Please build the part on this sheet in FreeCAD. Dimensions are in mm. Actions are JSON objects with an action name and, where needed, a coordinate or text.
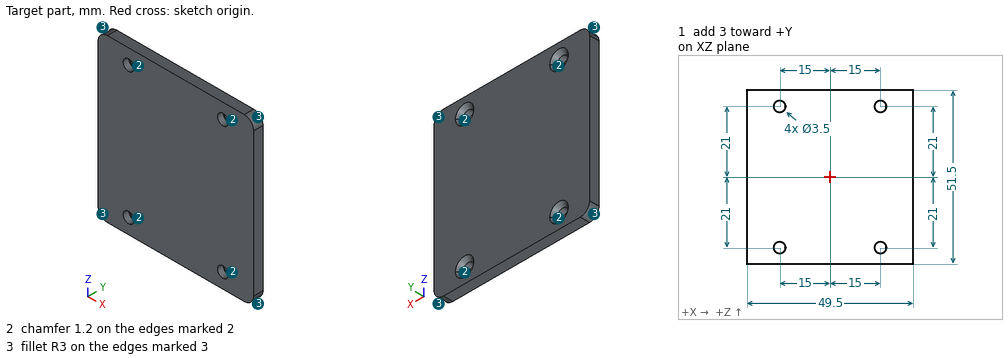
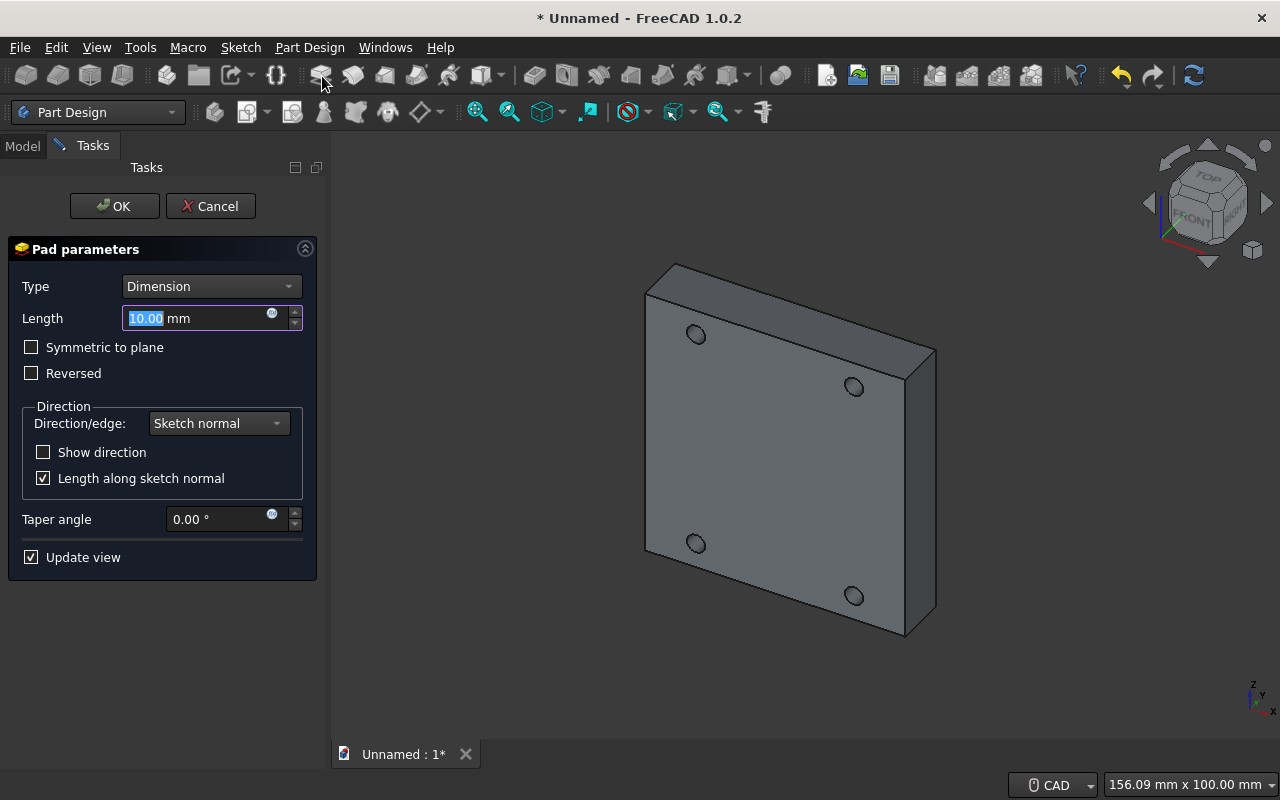
{"action": "type", "text": "3"}
{"action": "key", "text": "Tab"}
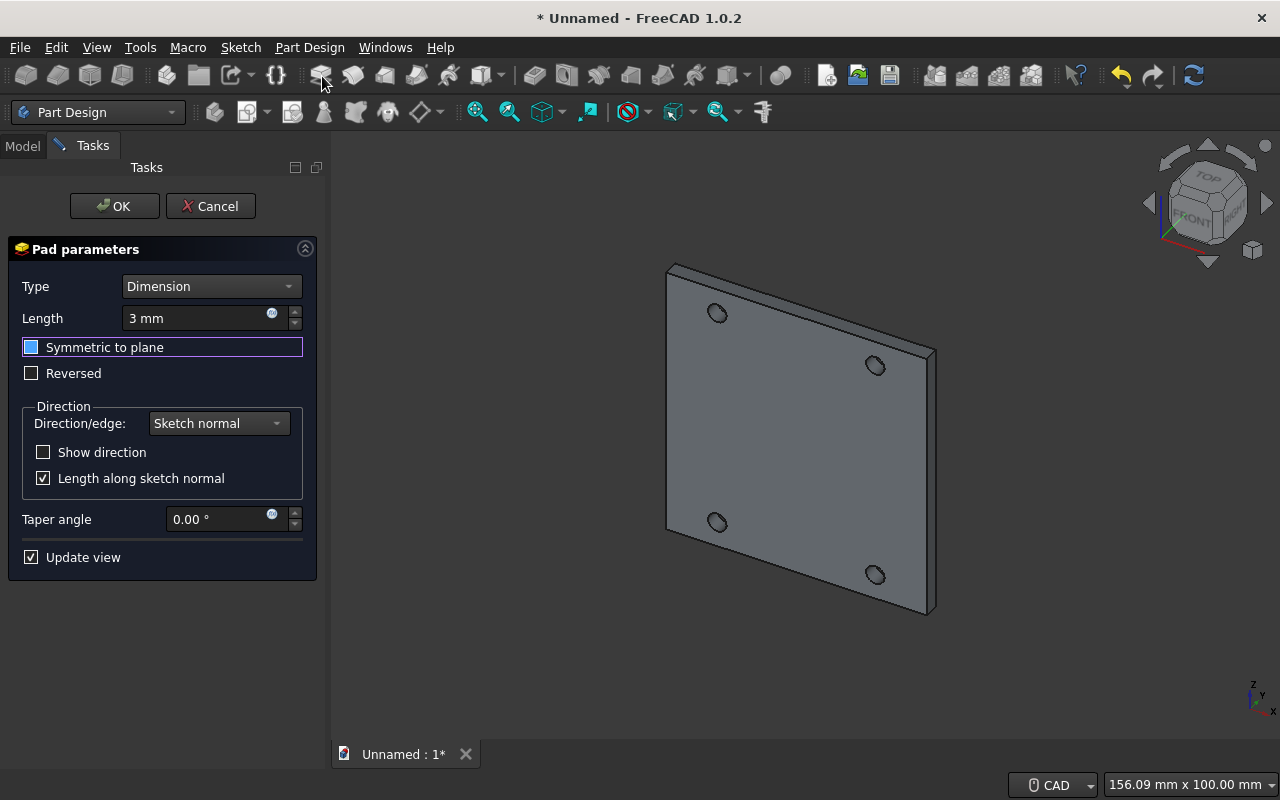
{"action": "left_click", "coordinate": [30, 373]}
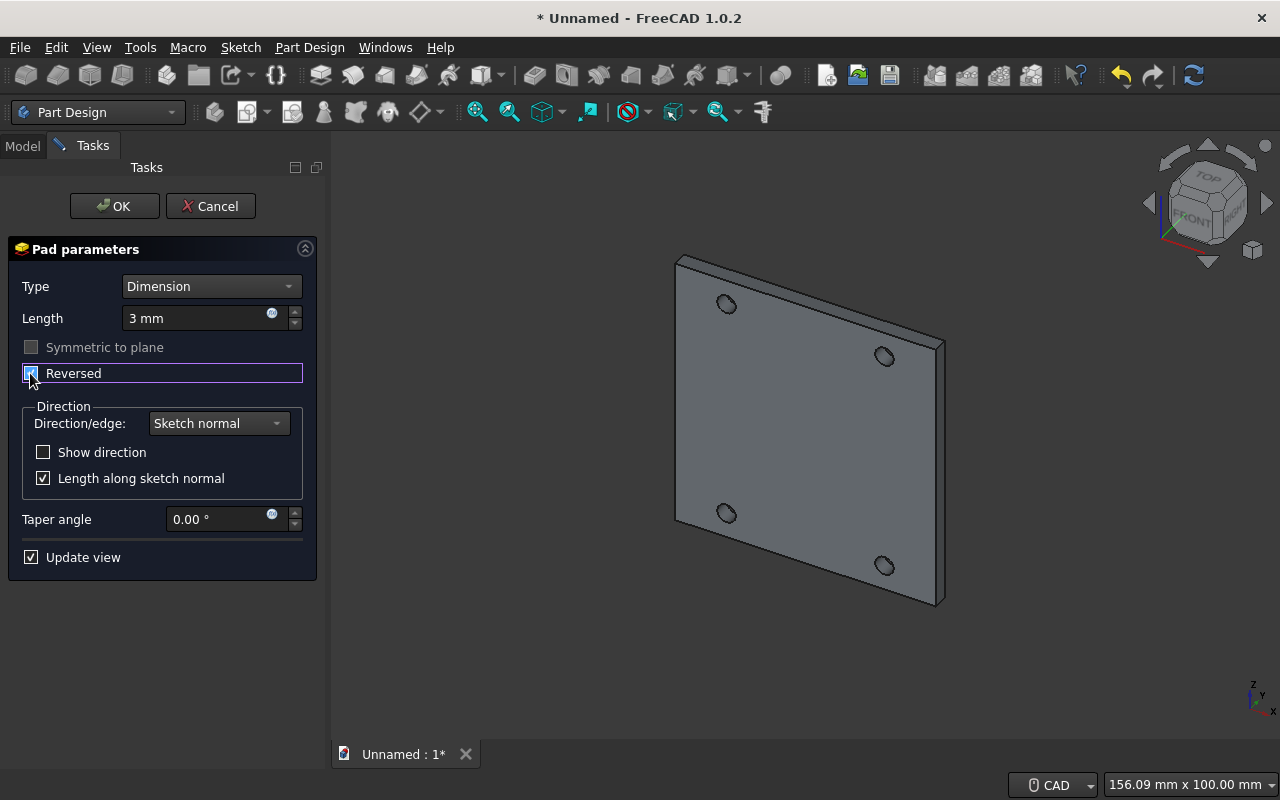
{"action": "left_click", "coordinate": [115, 206]}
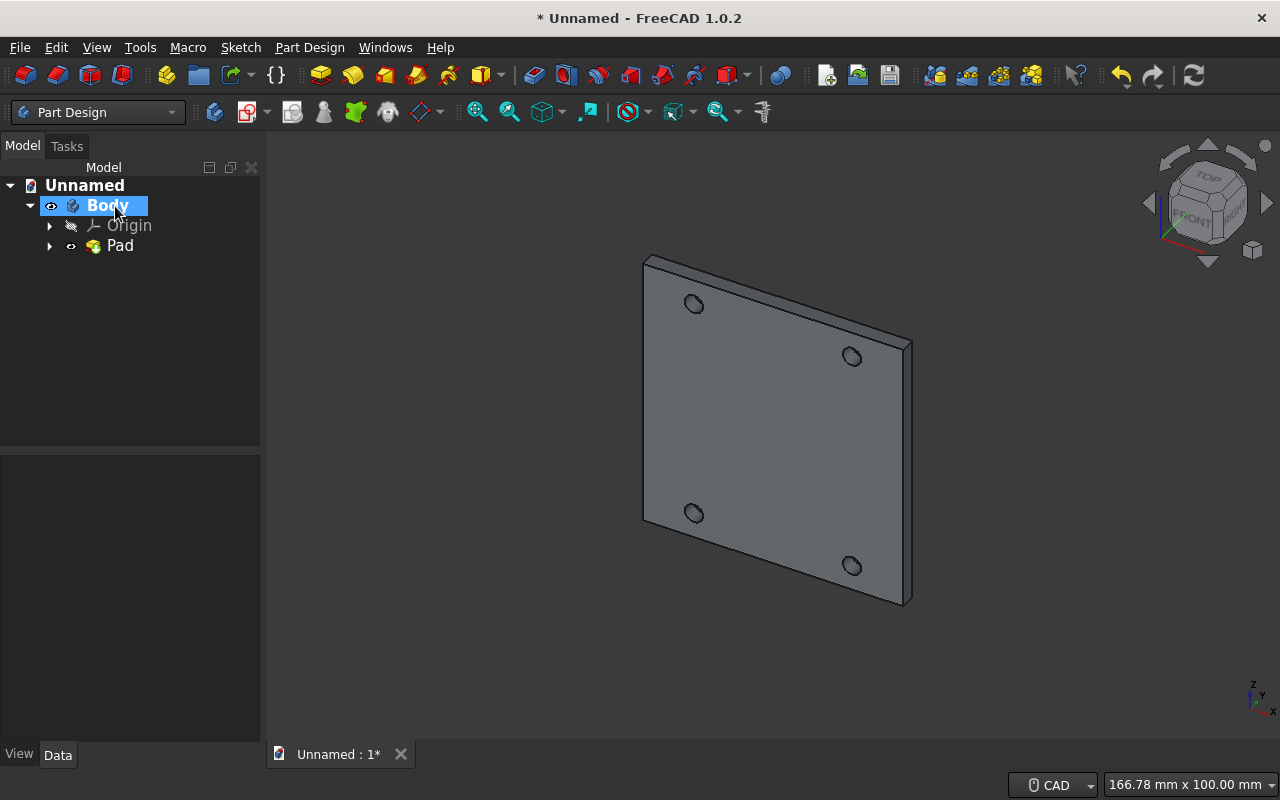
{"action": "key", "text": "0"}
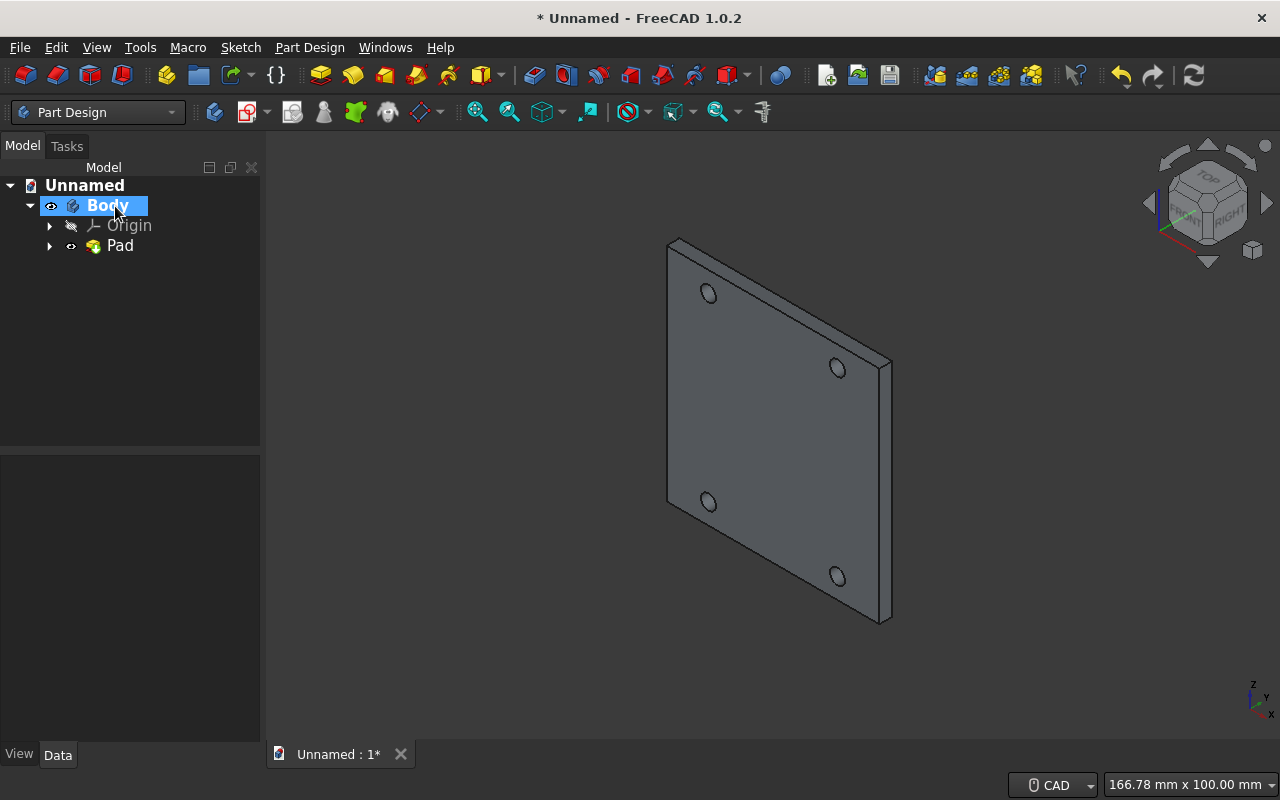
{"action": "key", "text": "2"}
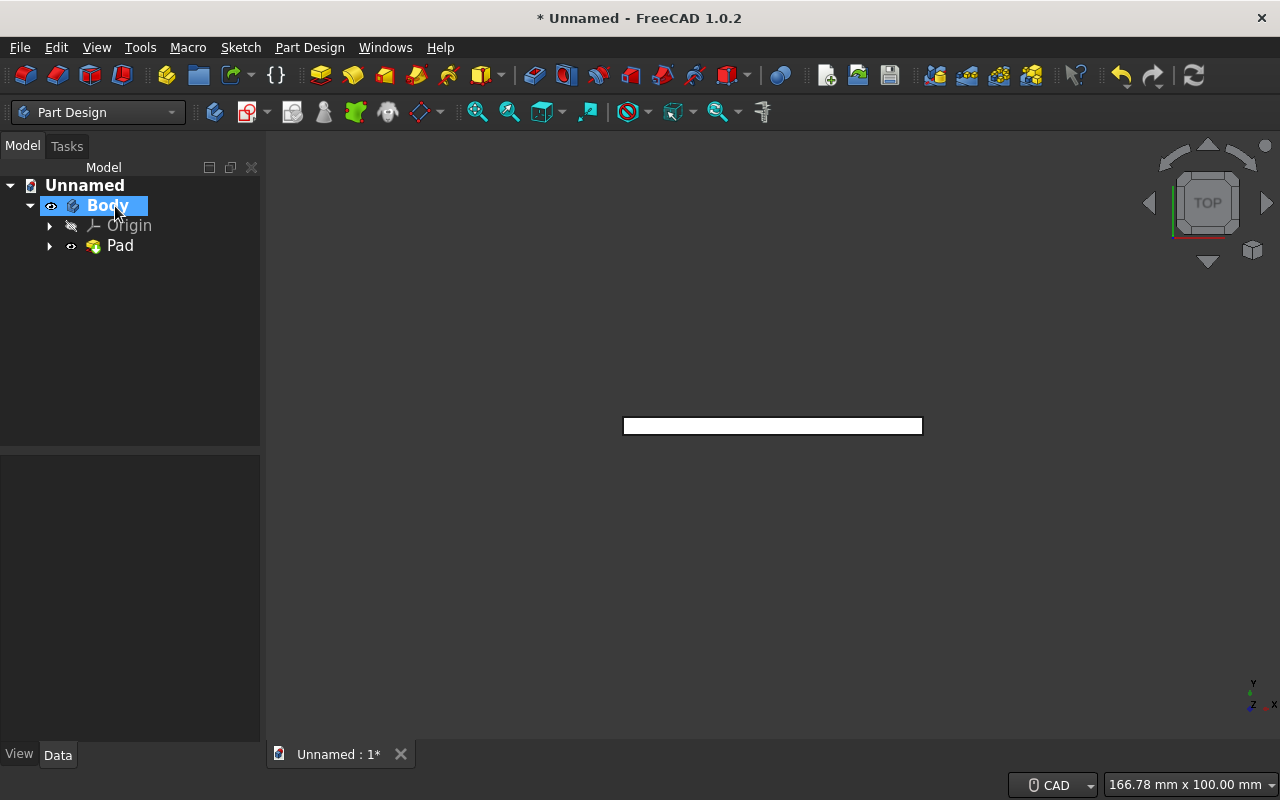
{"action": "left_click", "coordinate": [478, 112]}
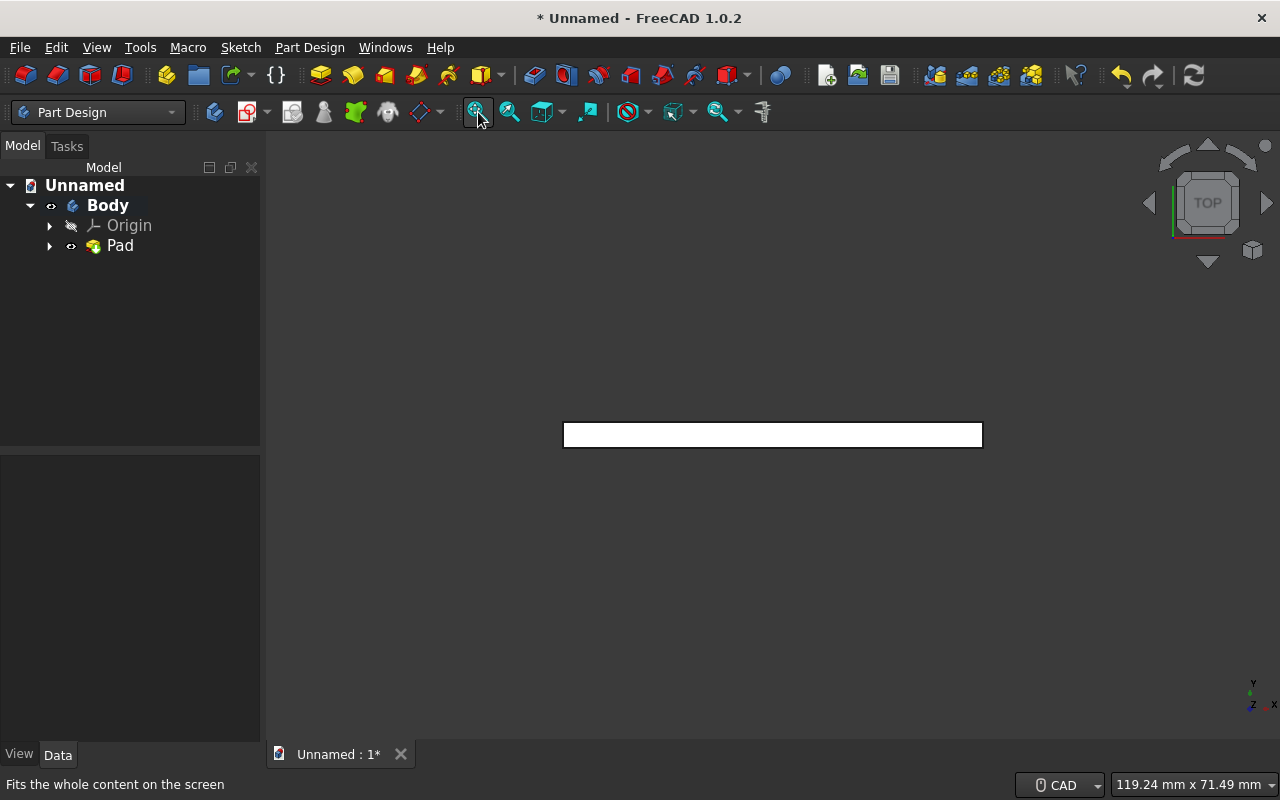
{"action": "key", "text": "1"}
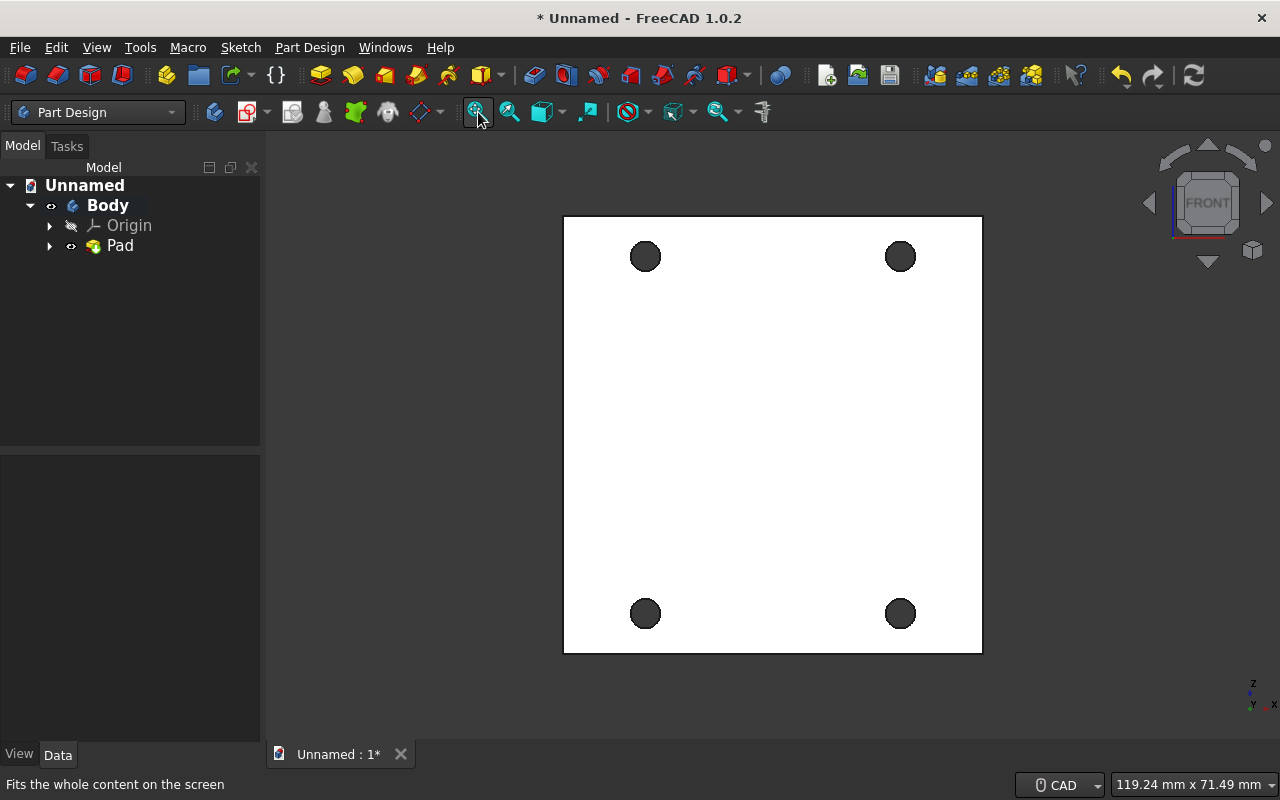
{"action": "key", "text": "3"}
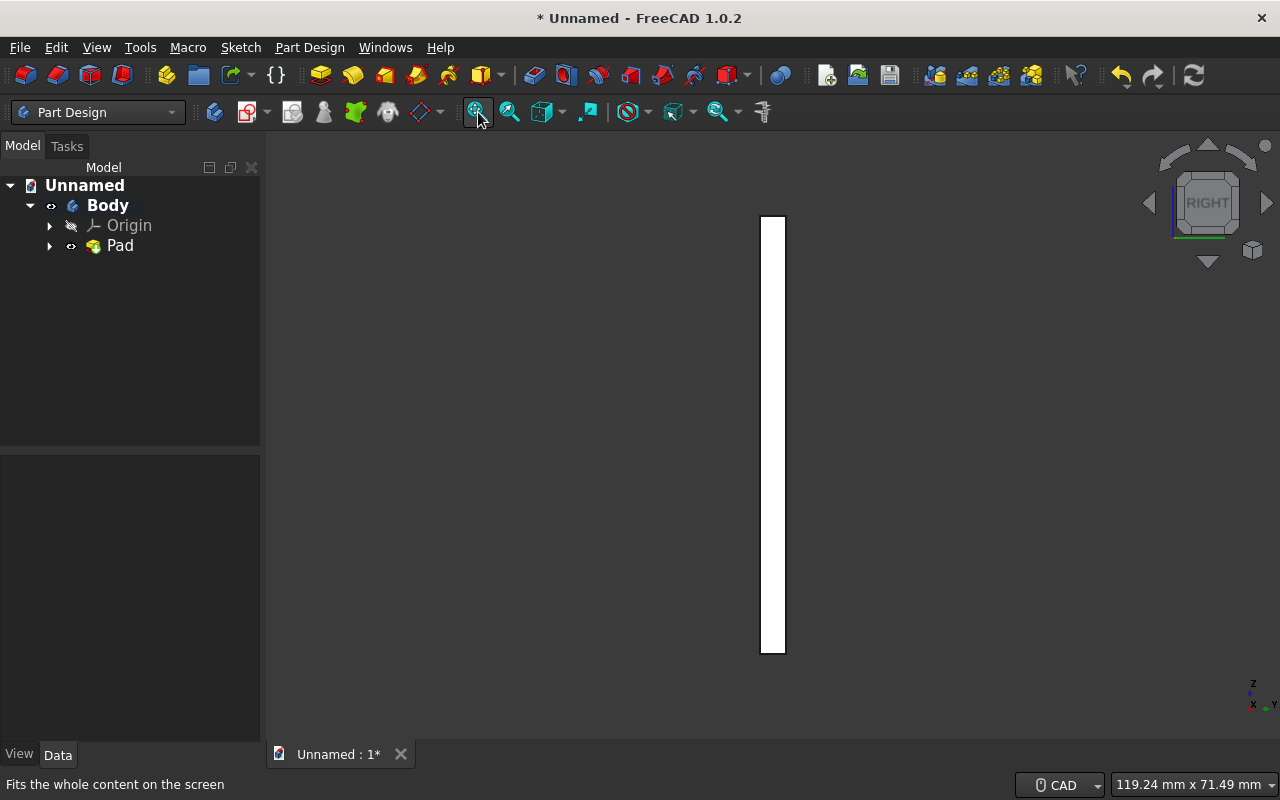
{"action": "key", "text": "5"}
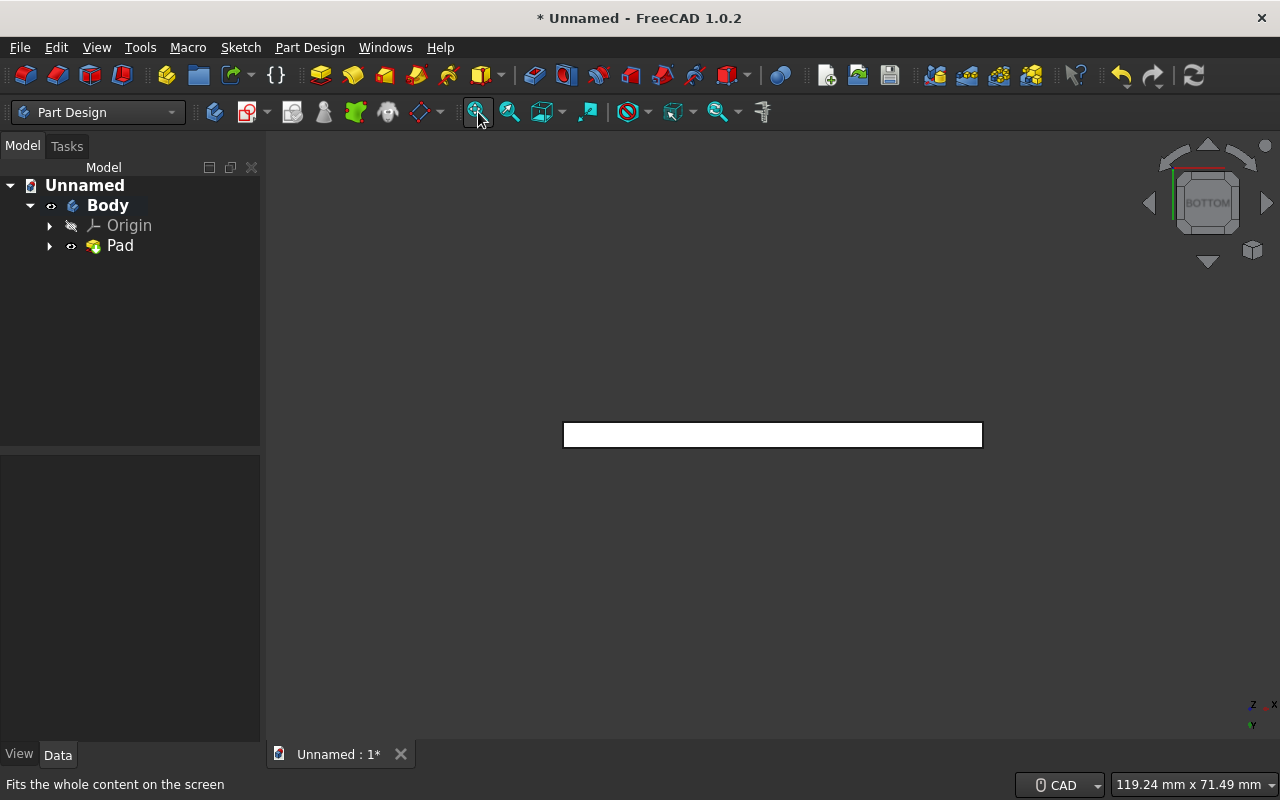
{"action": "left_click", "coordinate": [478, 112]}